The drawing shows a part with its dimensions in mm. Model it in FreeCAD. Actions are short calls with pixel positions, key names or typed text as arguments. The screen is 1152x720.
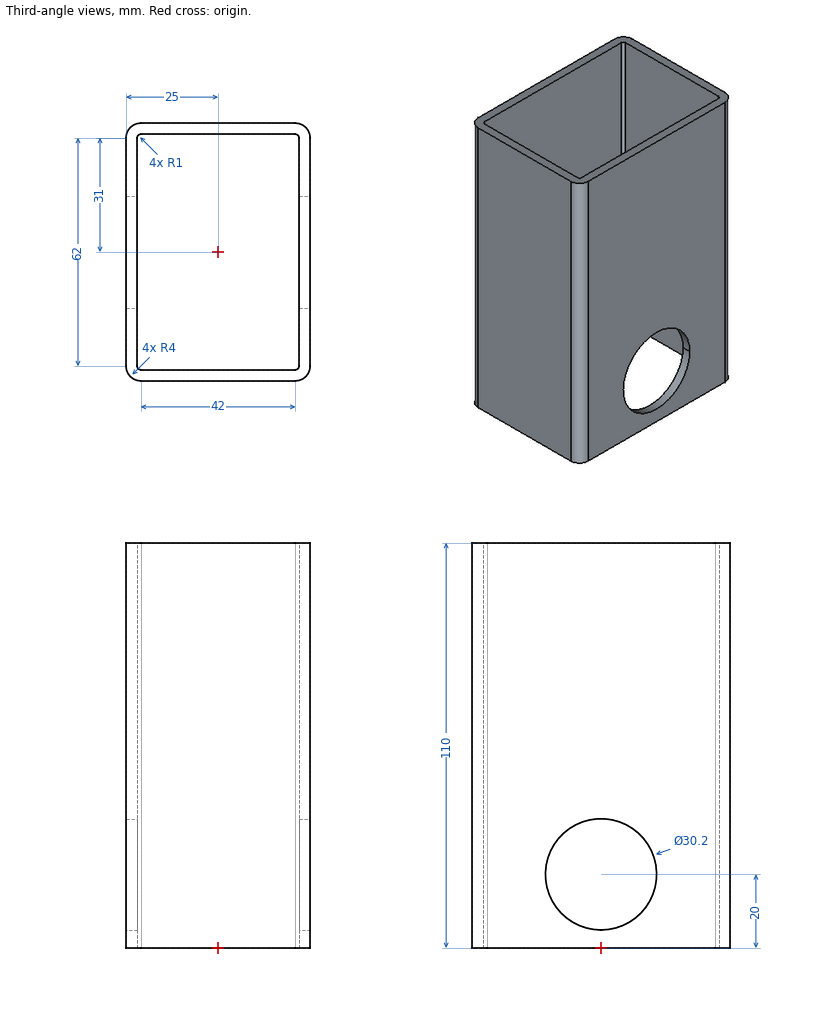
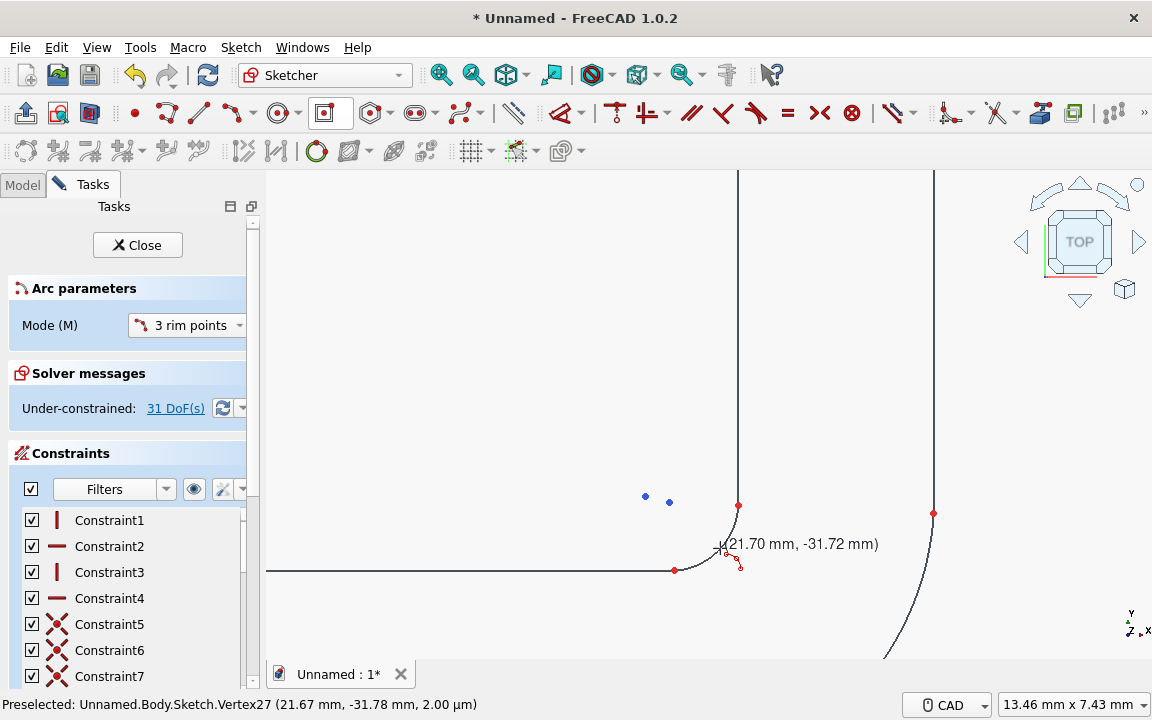
scroll(728, 541, down, 14)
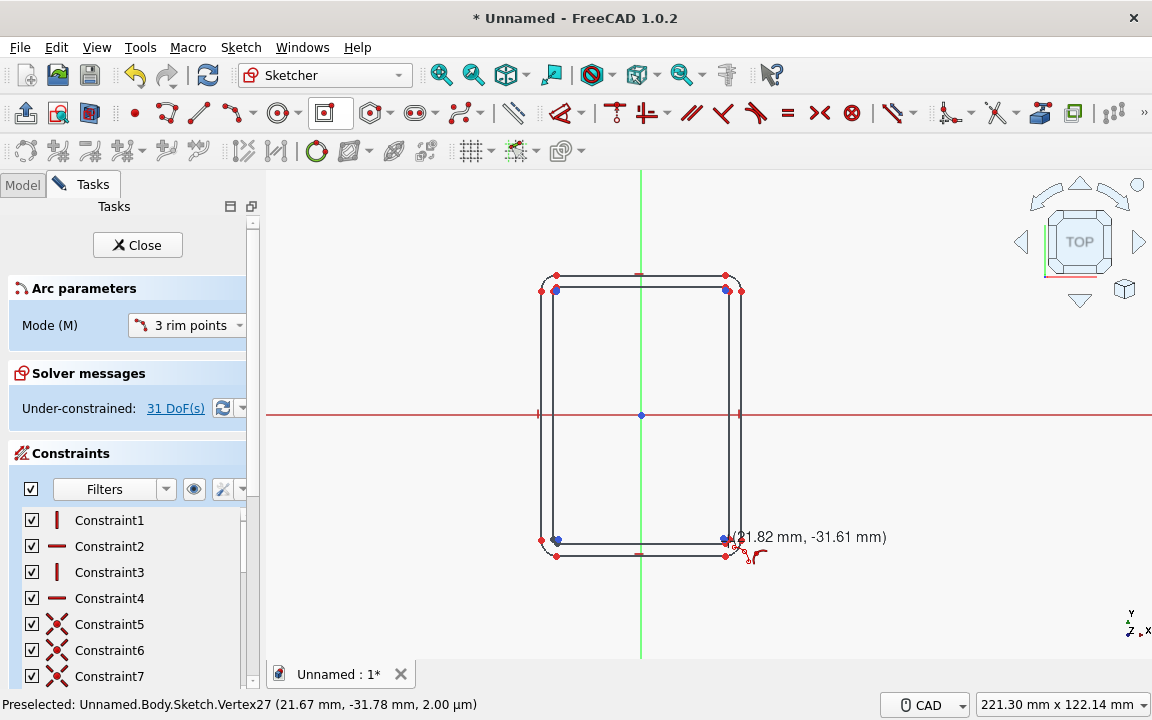
scroll(557, 543, up, 7)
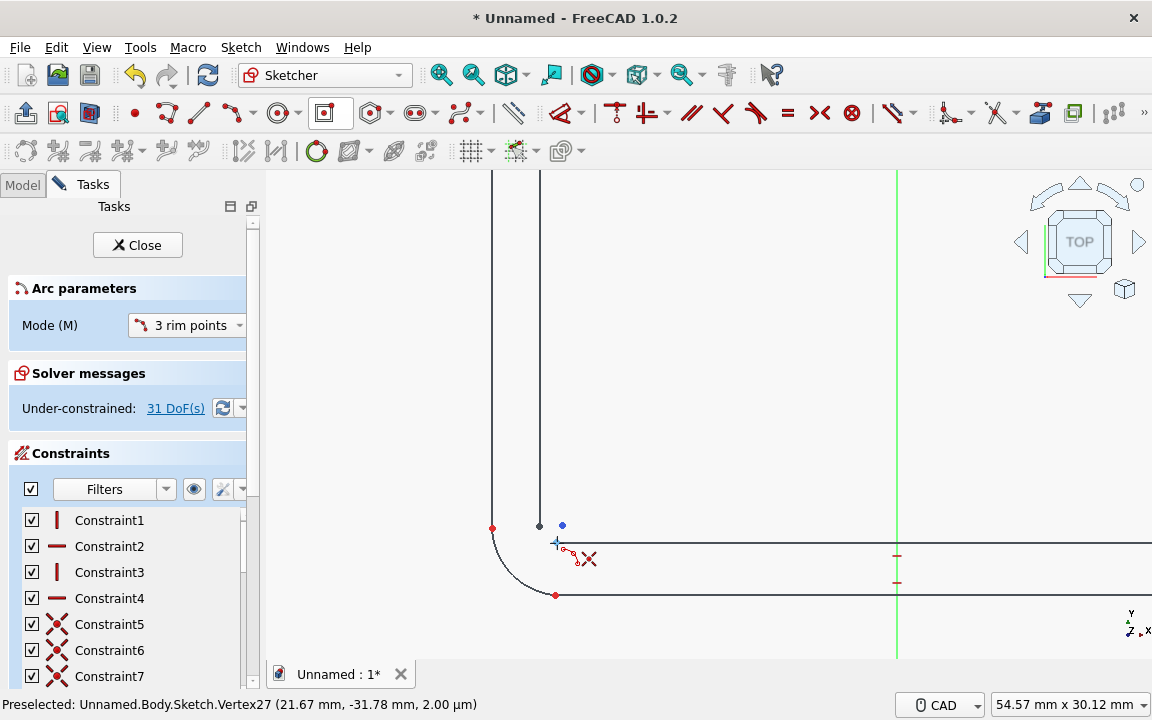
click(556, 543)
click(540, 527)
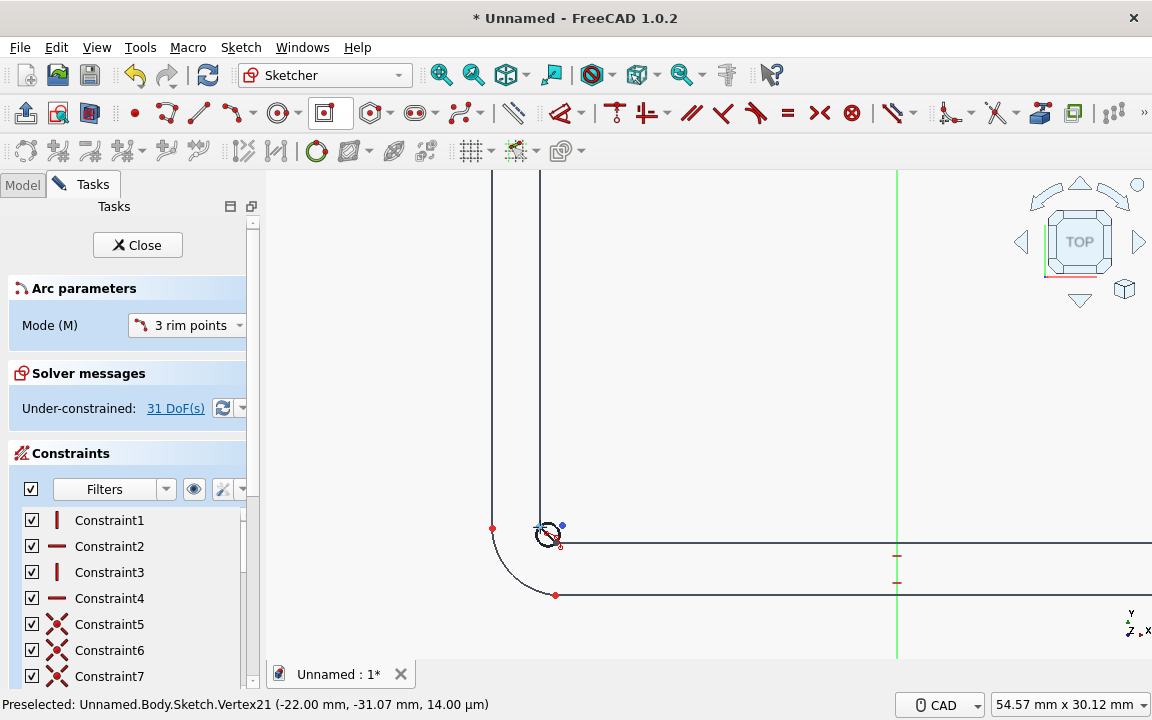
scroll(545, 537, up, 7)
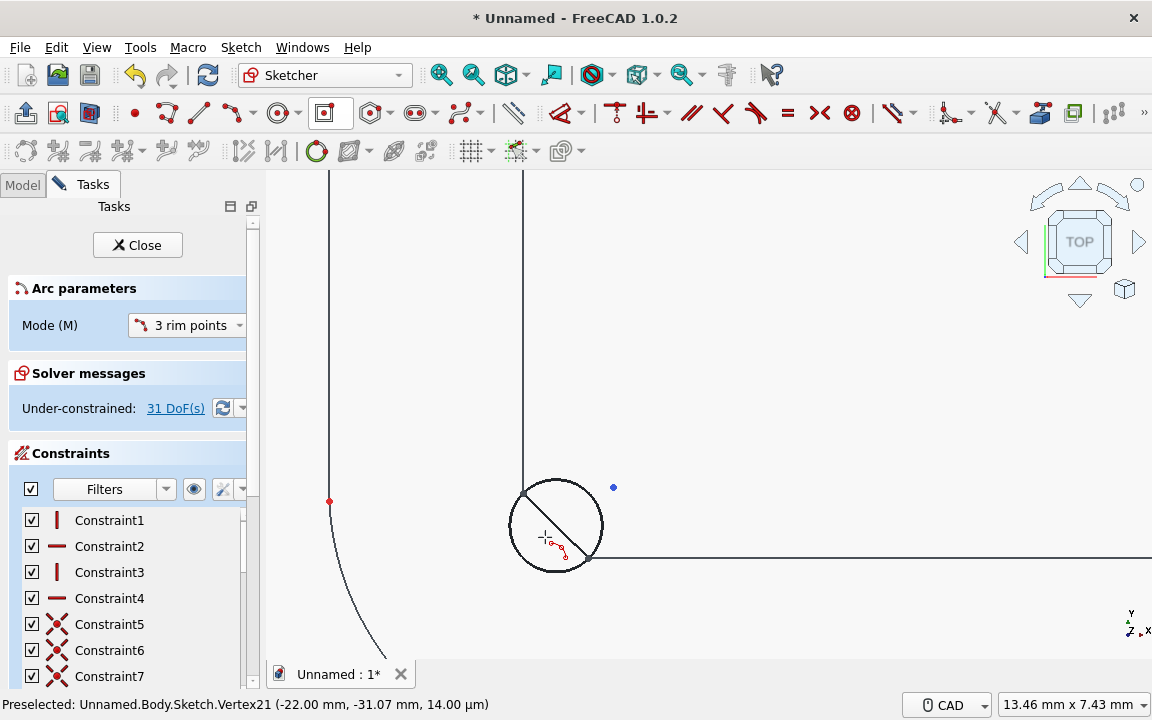
click(543, 536)
key(Escape)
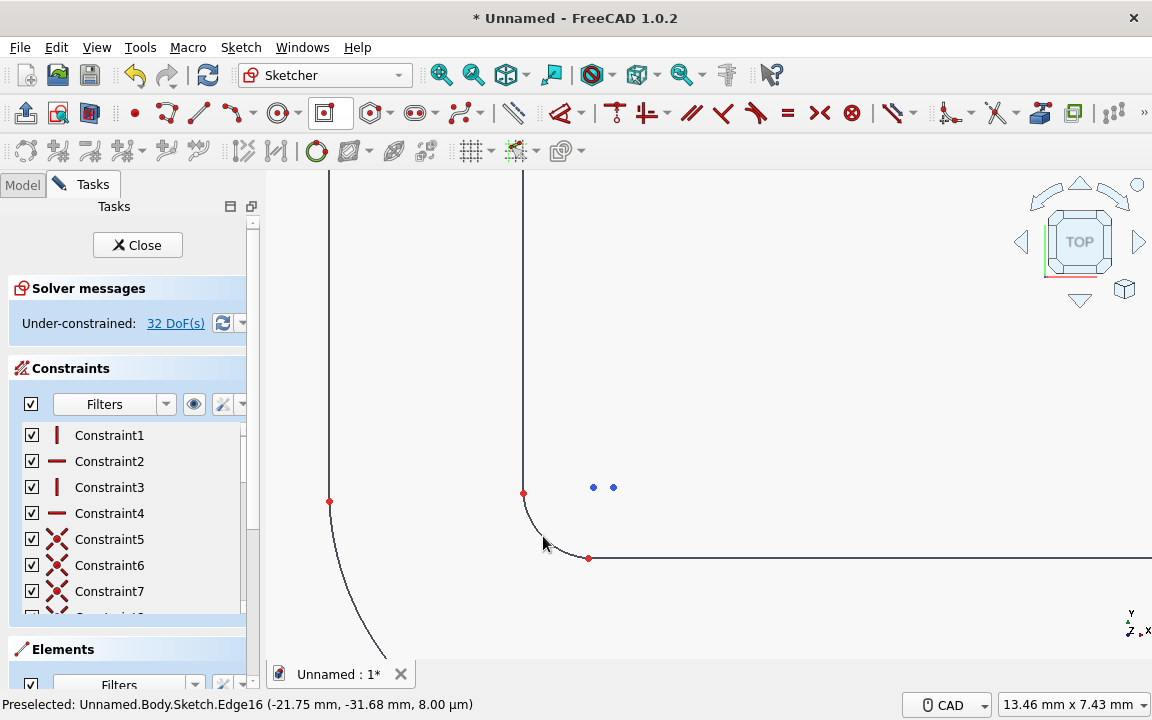
scroll(554, 542, down, 14)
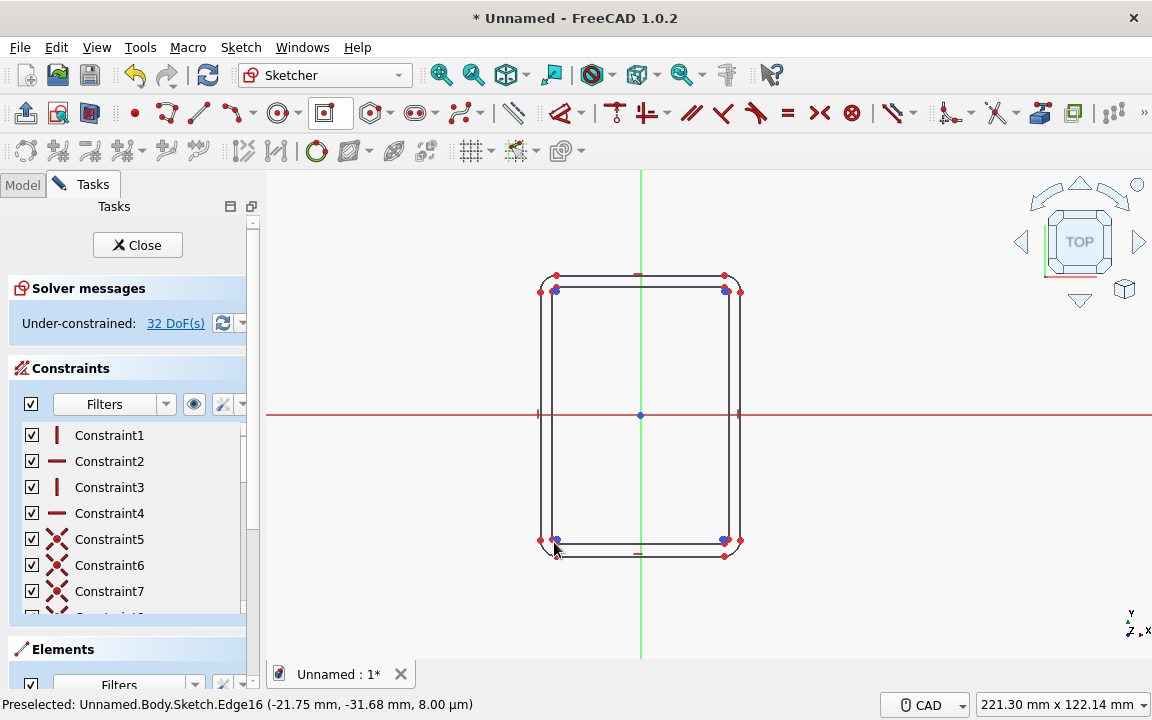
click(541, 367)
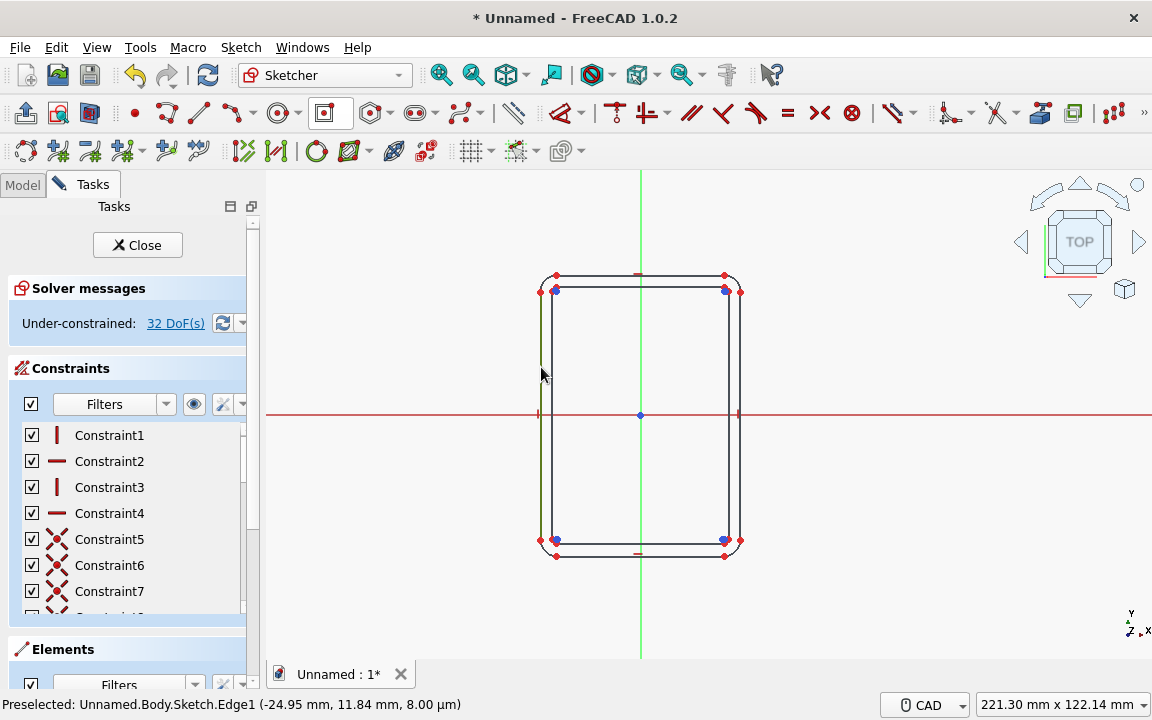
click(545, 551)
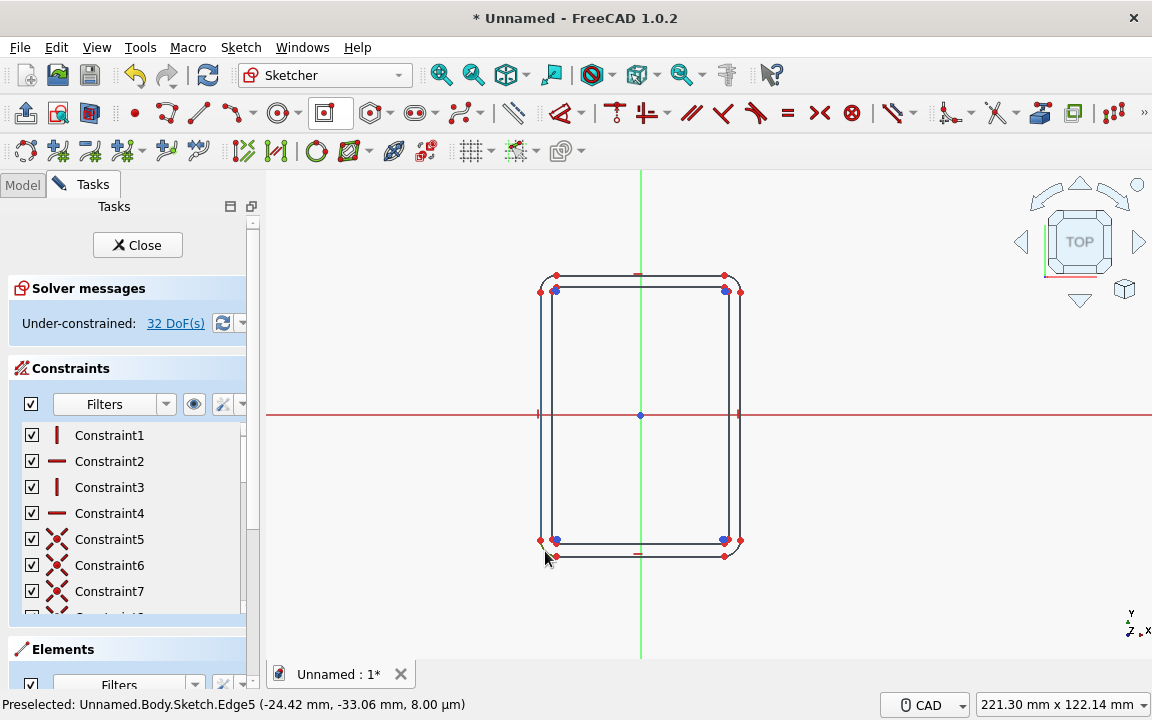
key(t)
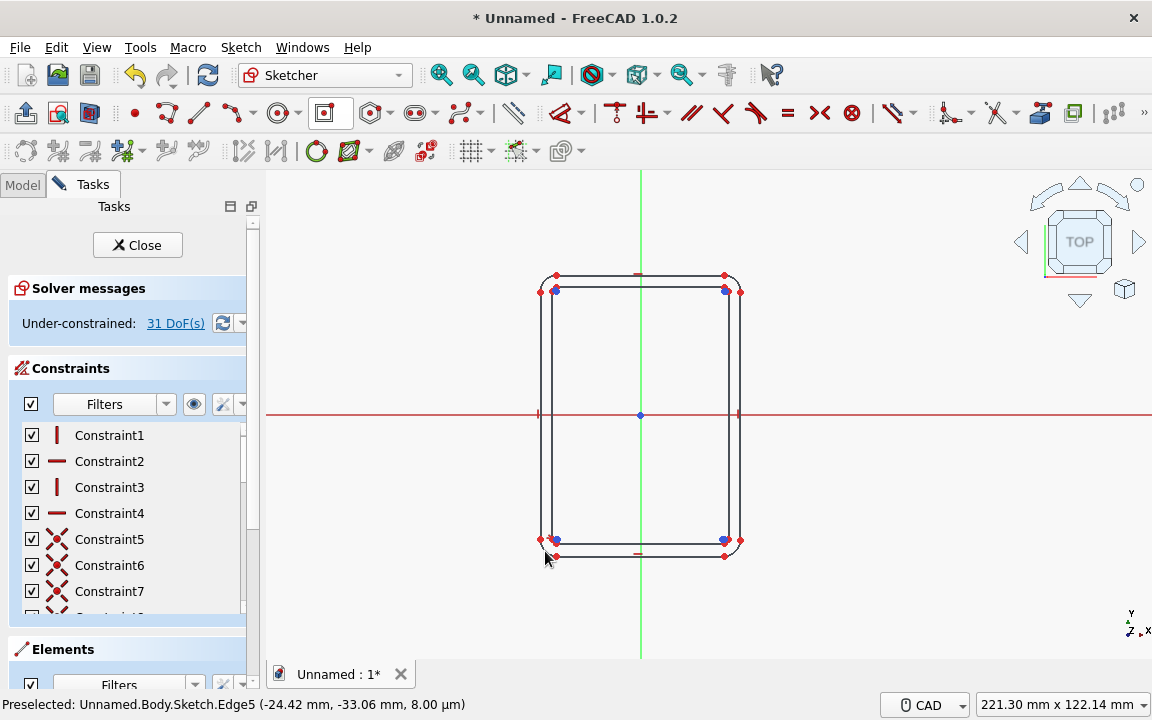
click(541, 366)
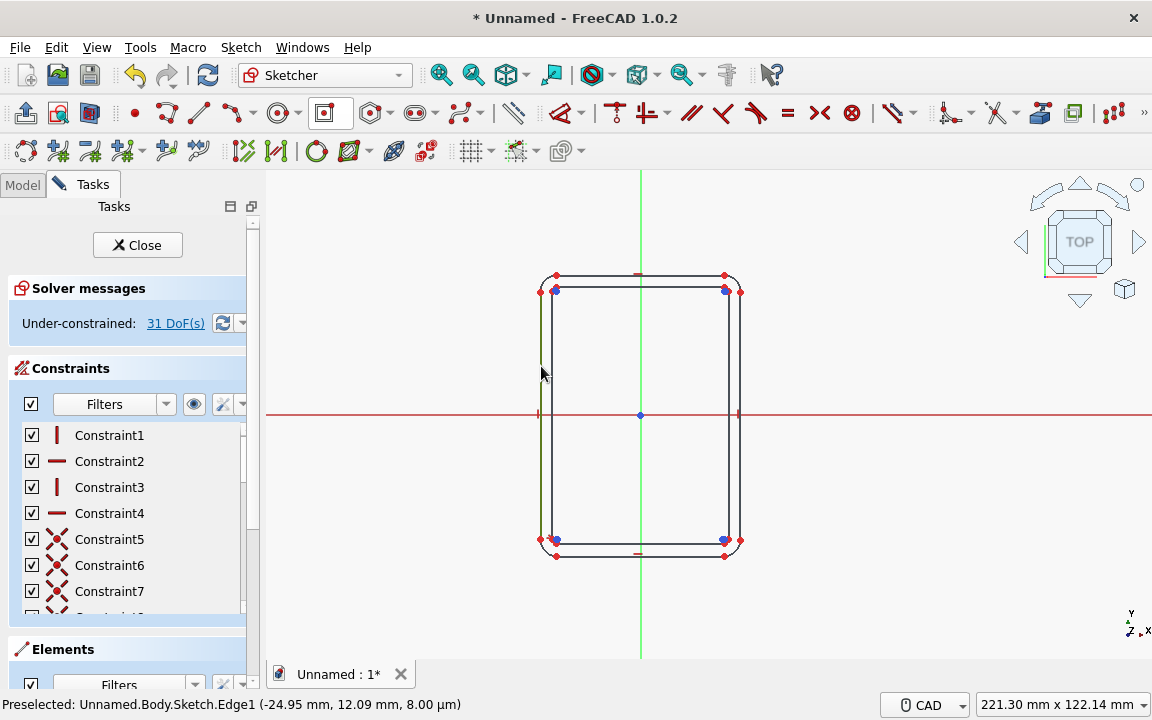
click(545, 281)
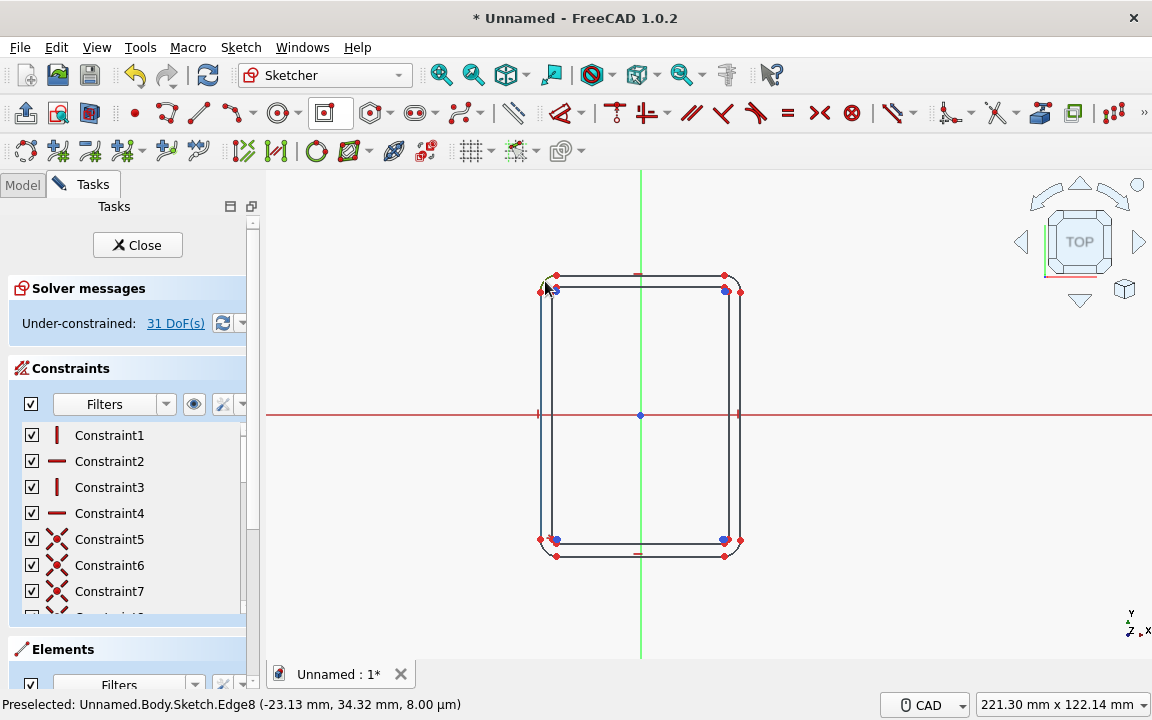
click(756, 114)